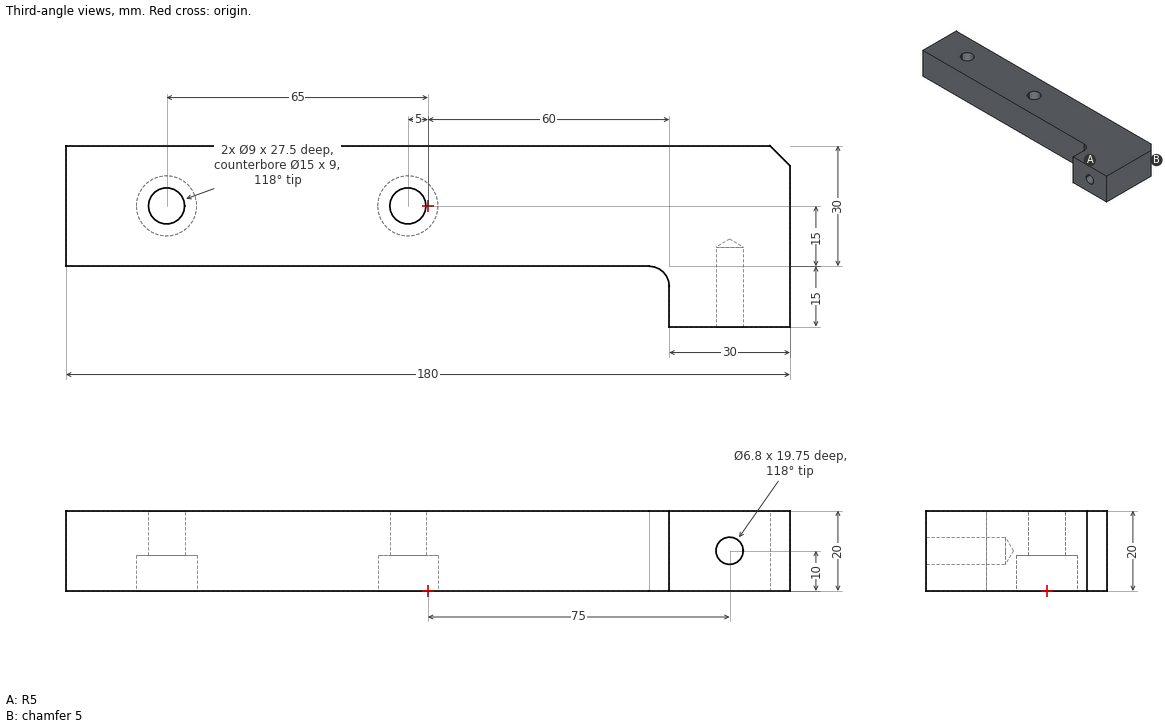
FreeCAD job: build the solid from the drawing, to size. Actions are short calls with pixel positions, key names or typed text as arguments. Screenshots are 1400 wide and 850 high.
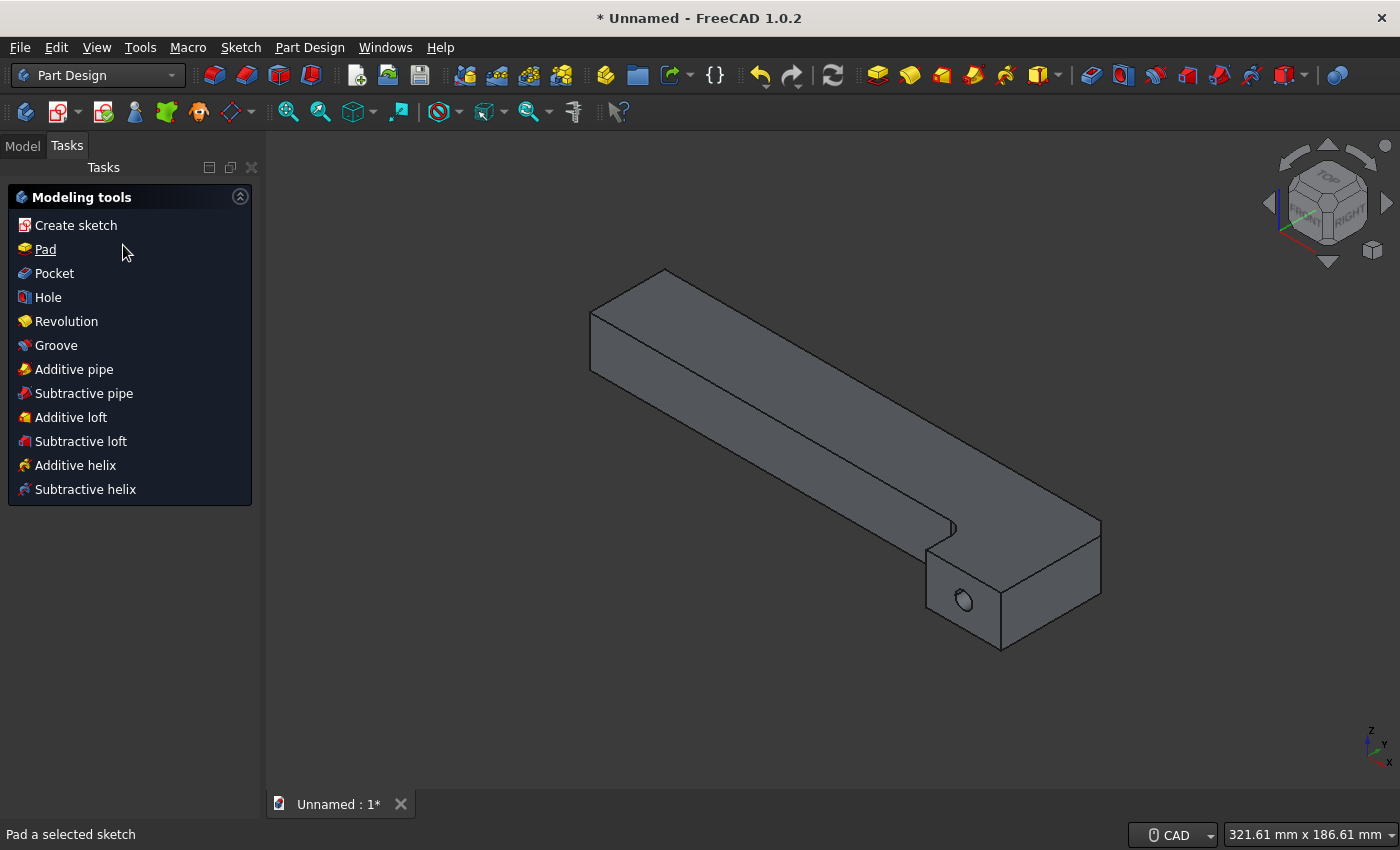
click(1124, 76)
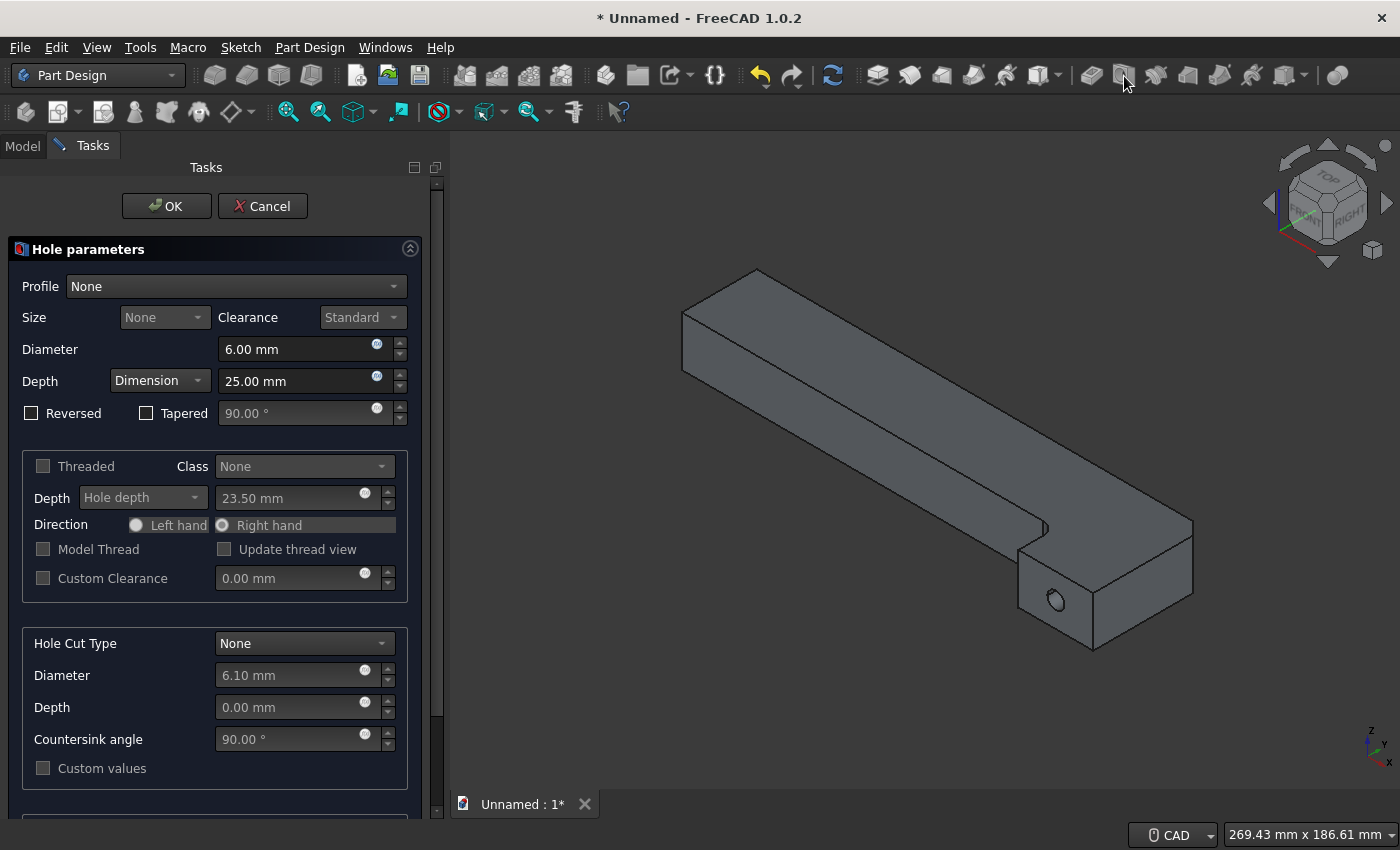
triple_click(305, 349)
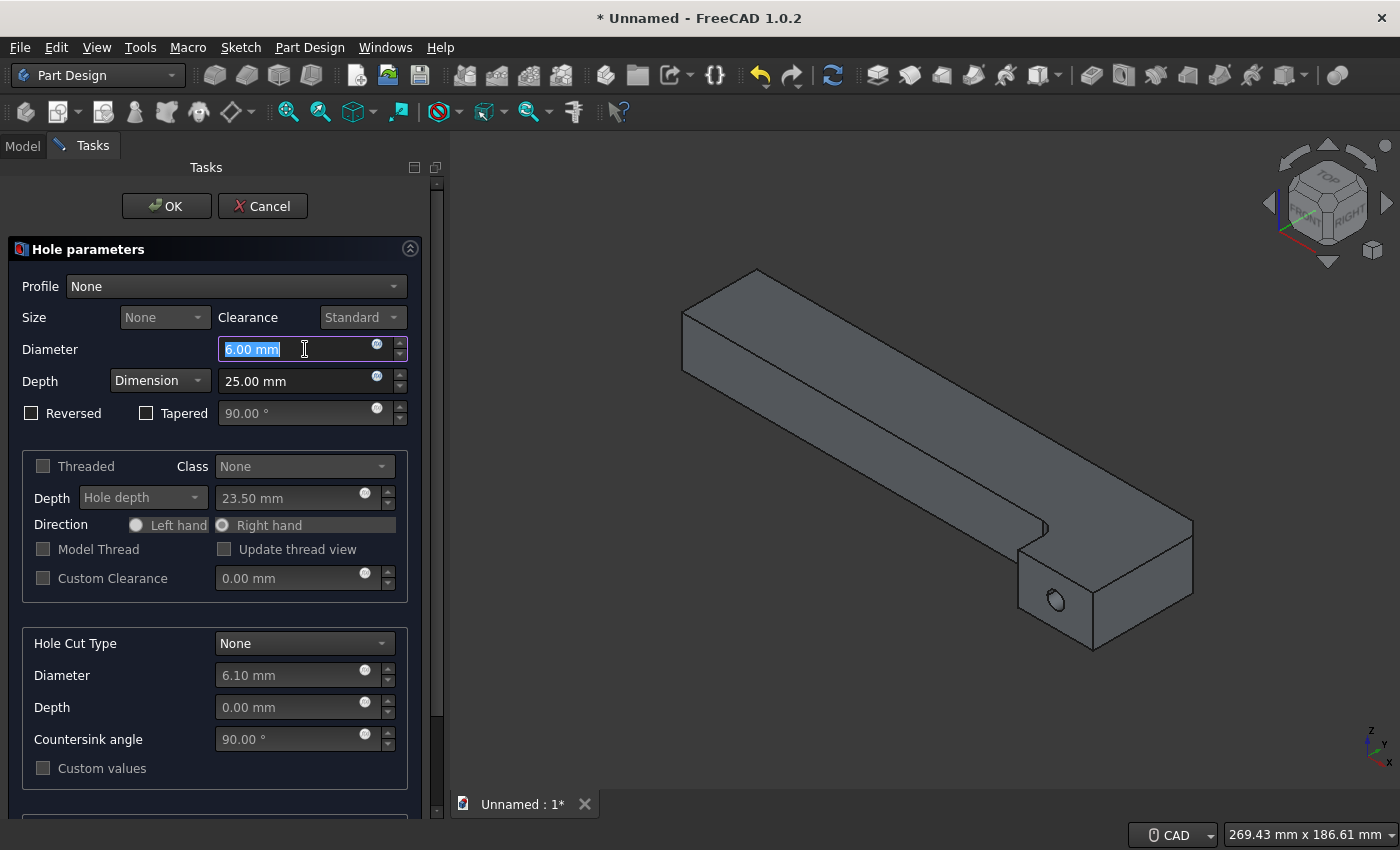
text(9)
key(Tab)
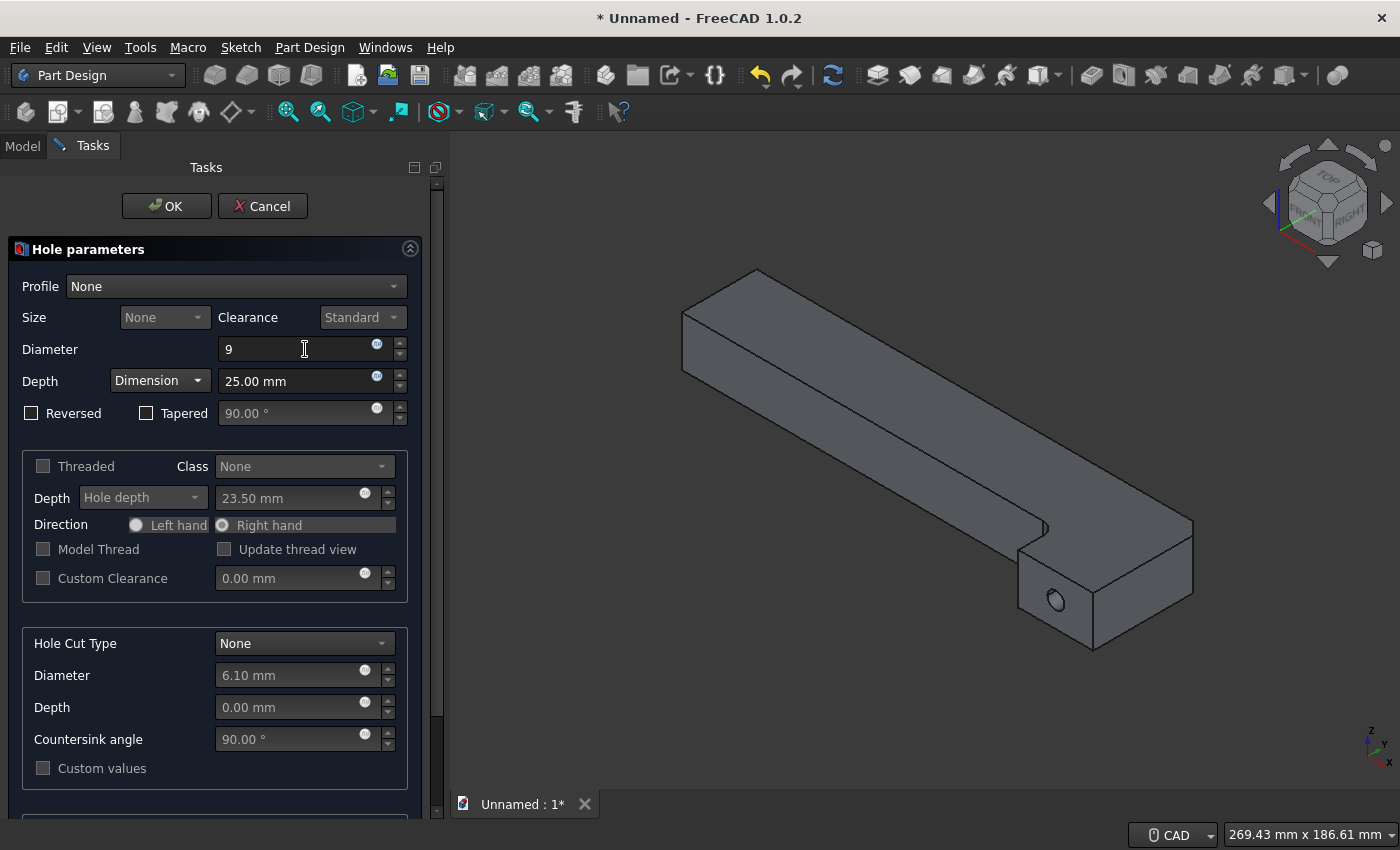
triple_click(305, 381)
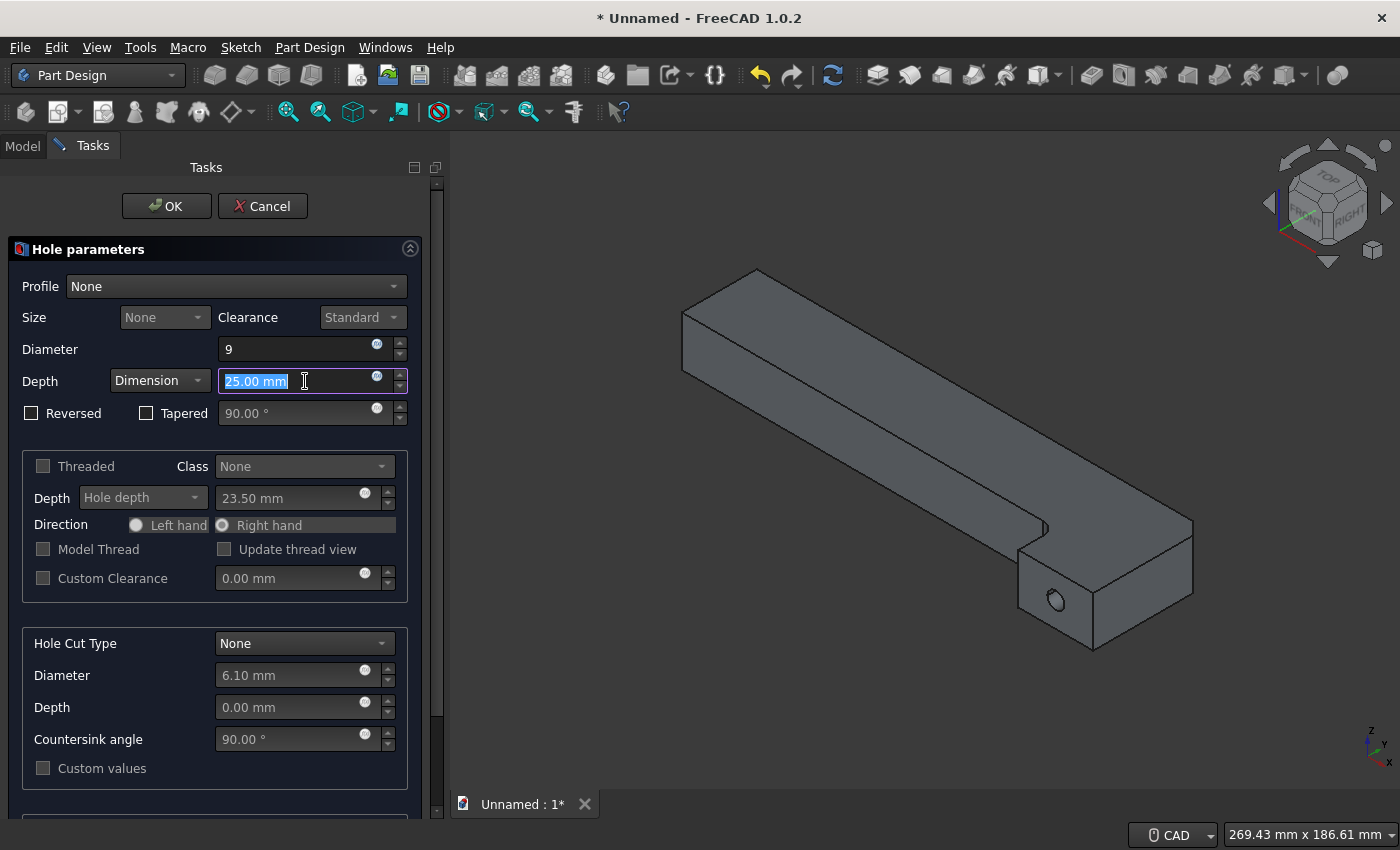
text(27.5)
key(Tab)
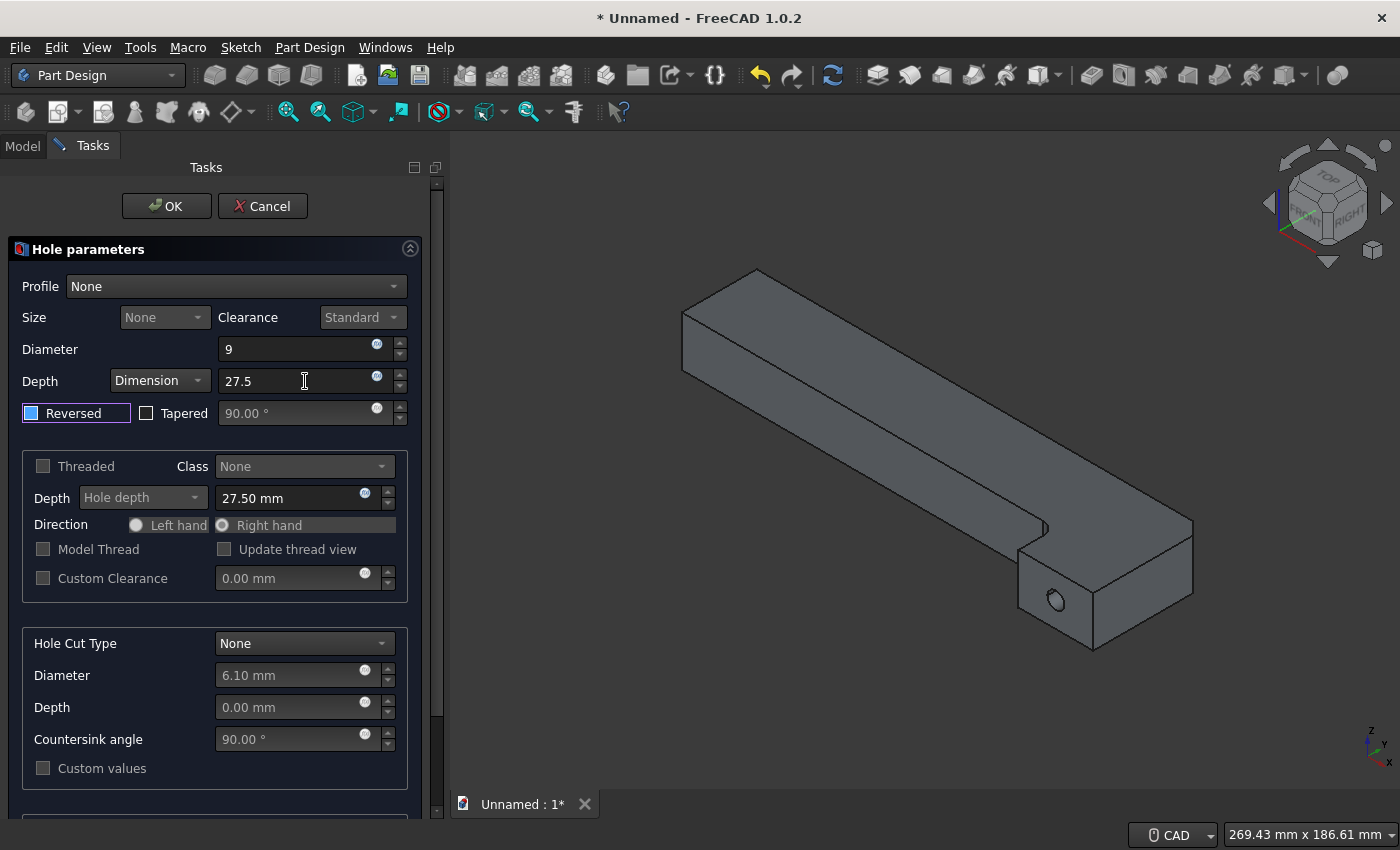
click(30, 413)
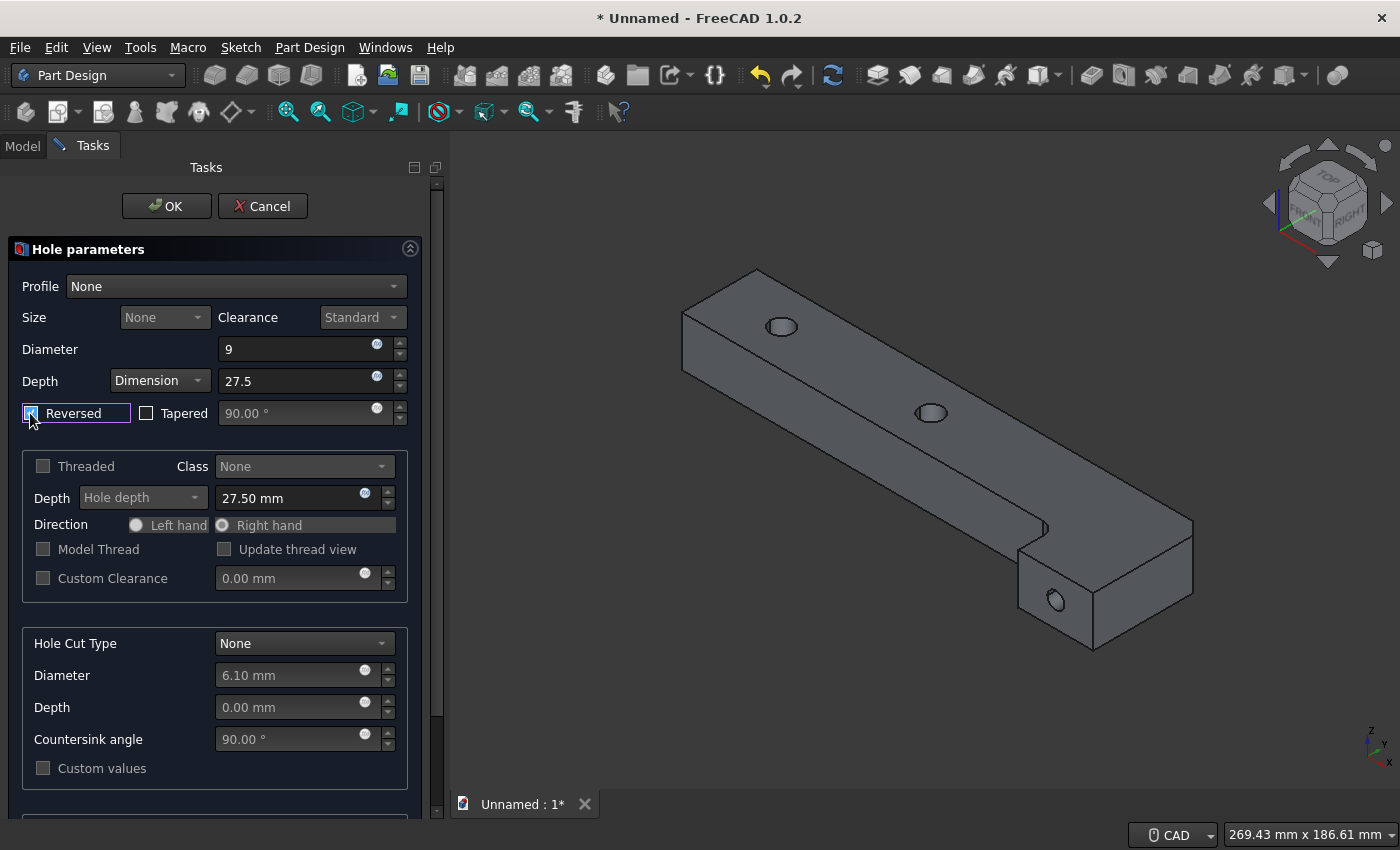
click(306, 644)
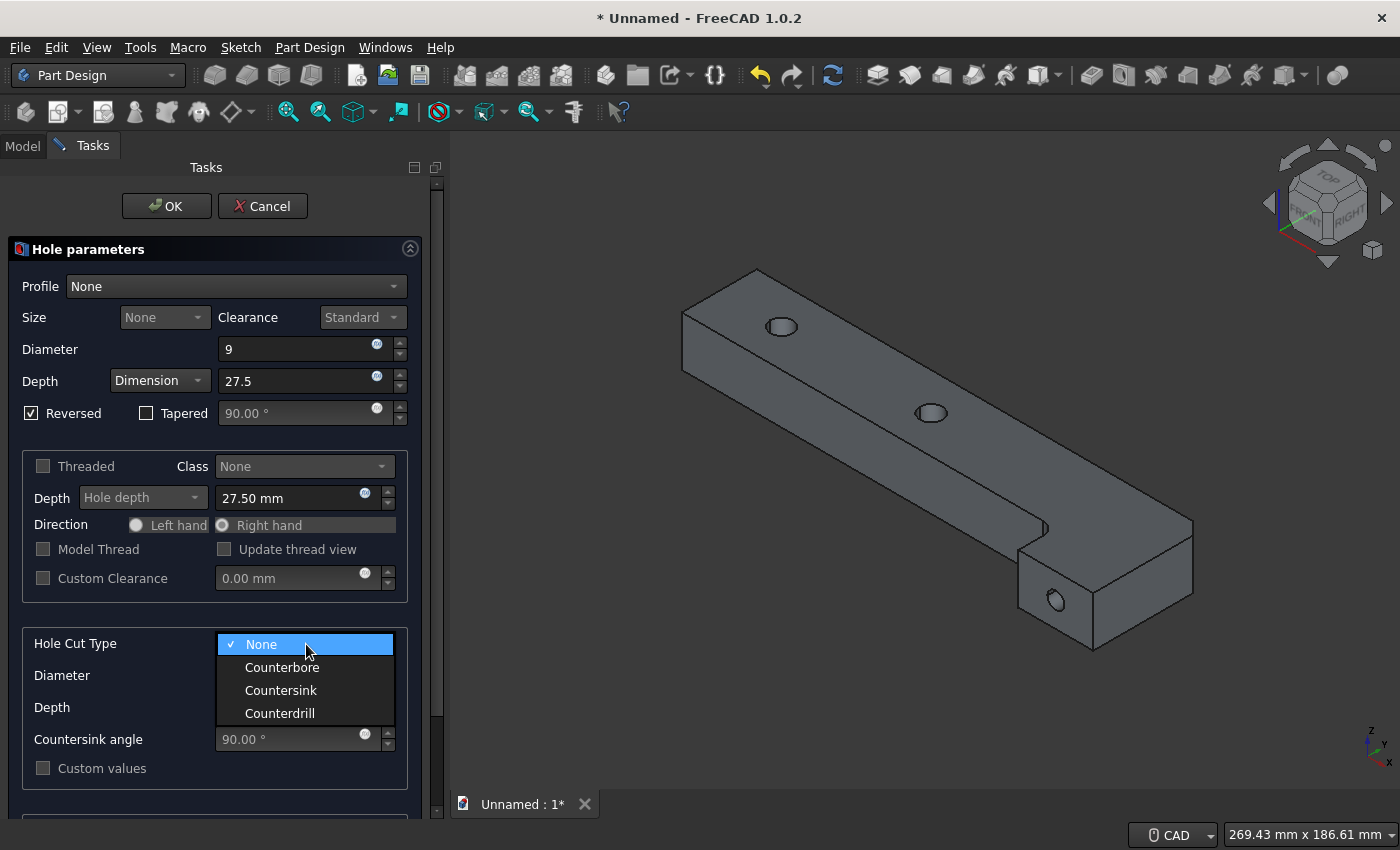
click(304, 668)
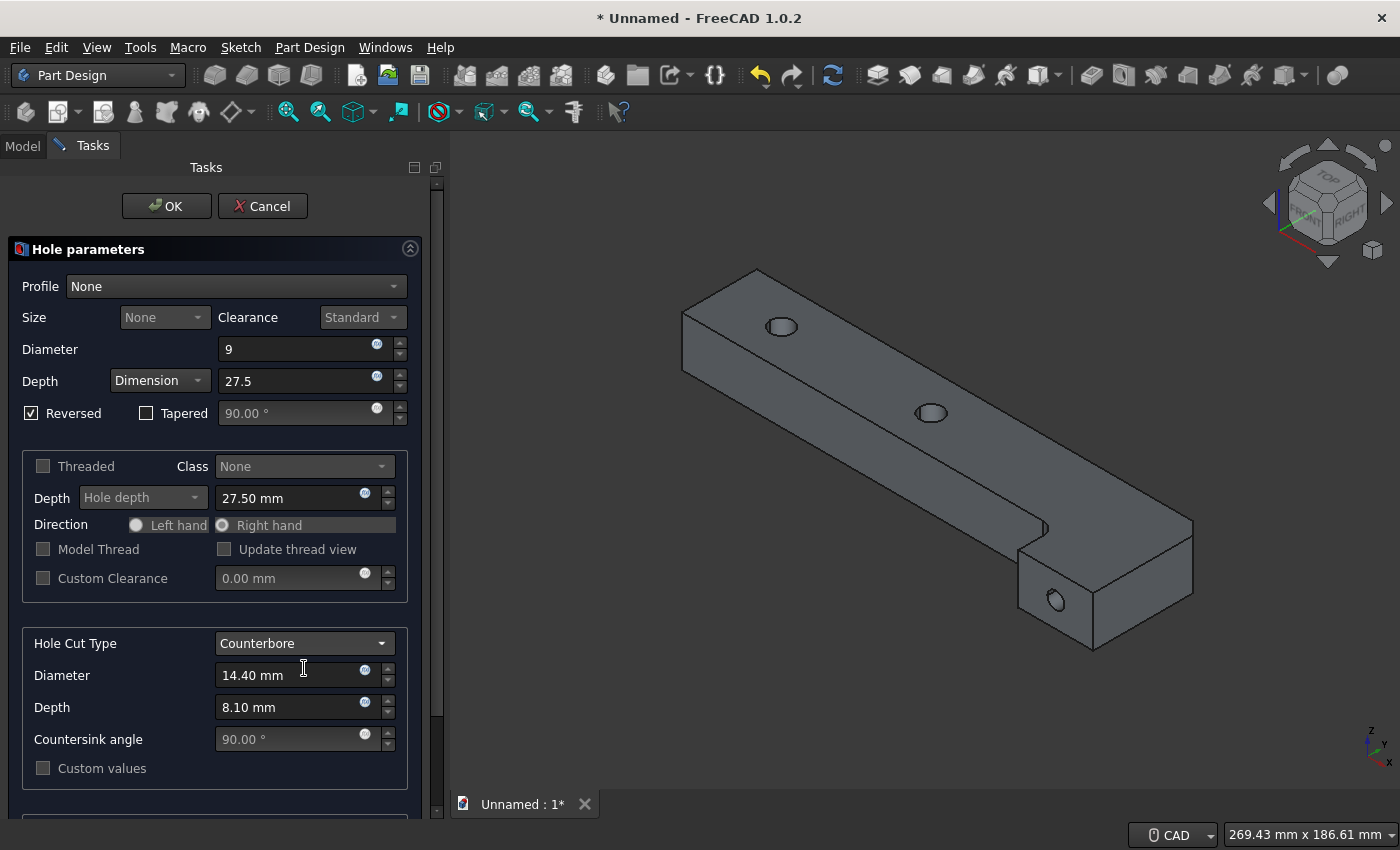
triple_click(298, 675)